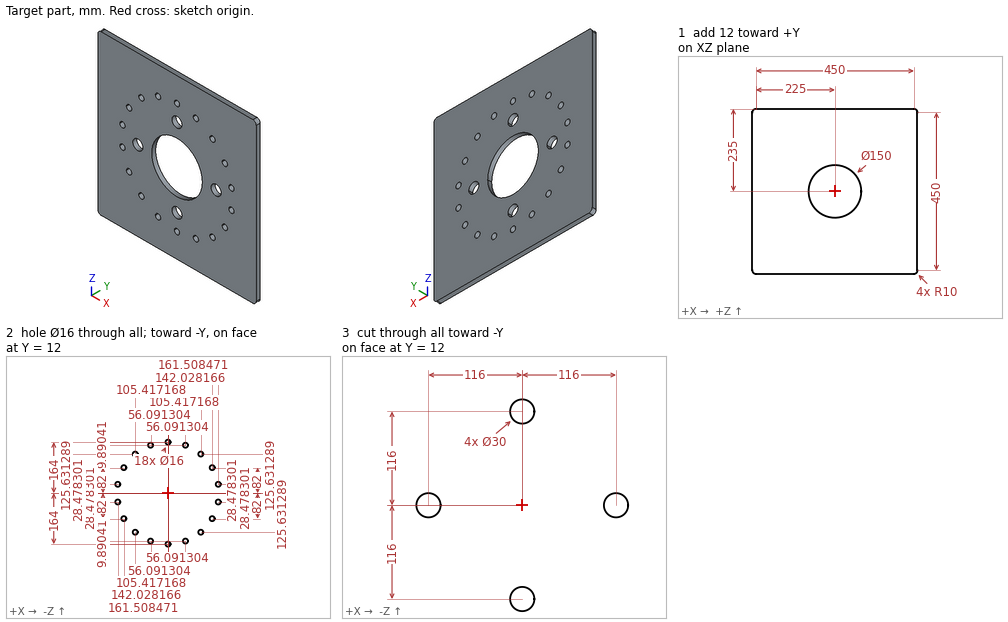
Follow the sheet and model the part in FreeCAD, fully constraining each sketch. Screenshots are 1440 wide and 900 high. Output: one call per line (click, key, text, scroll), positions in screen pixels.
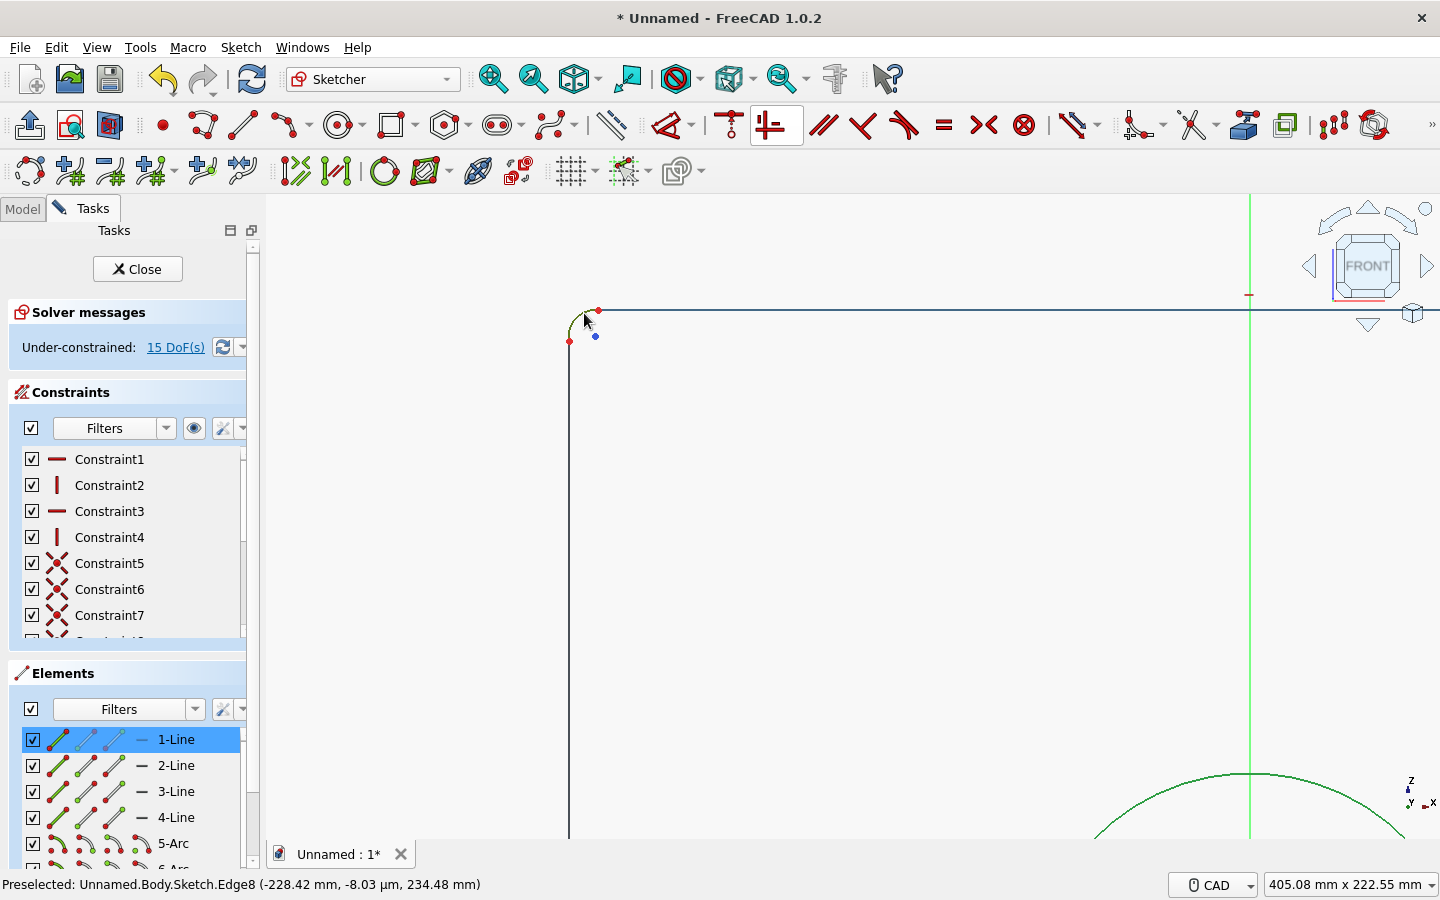
key(t)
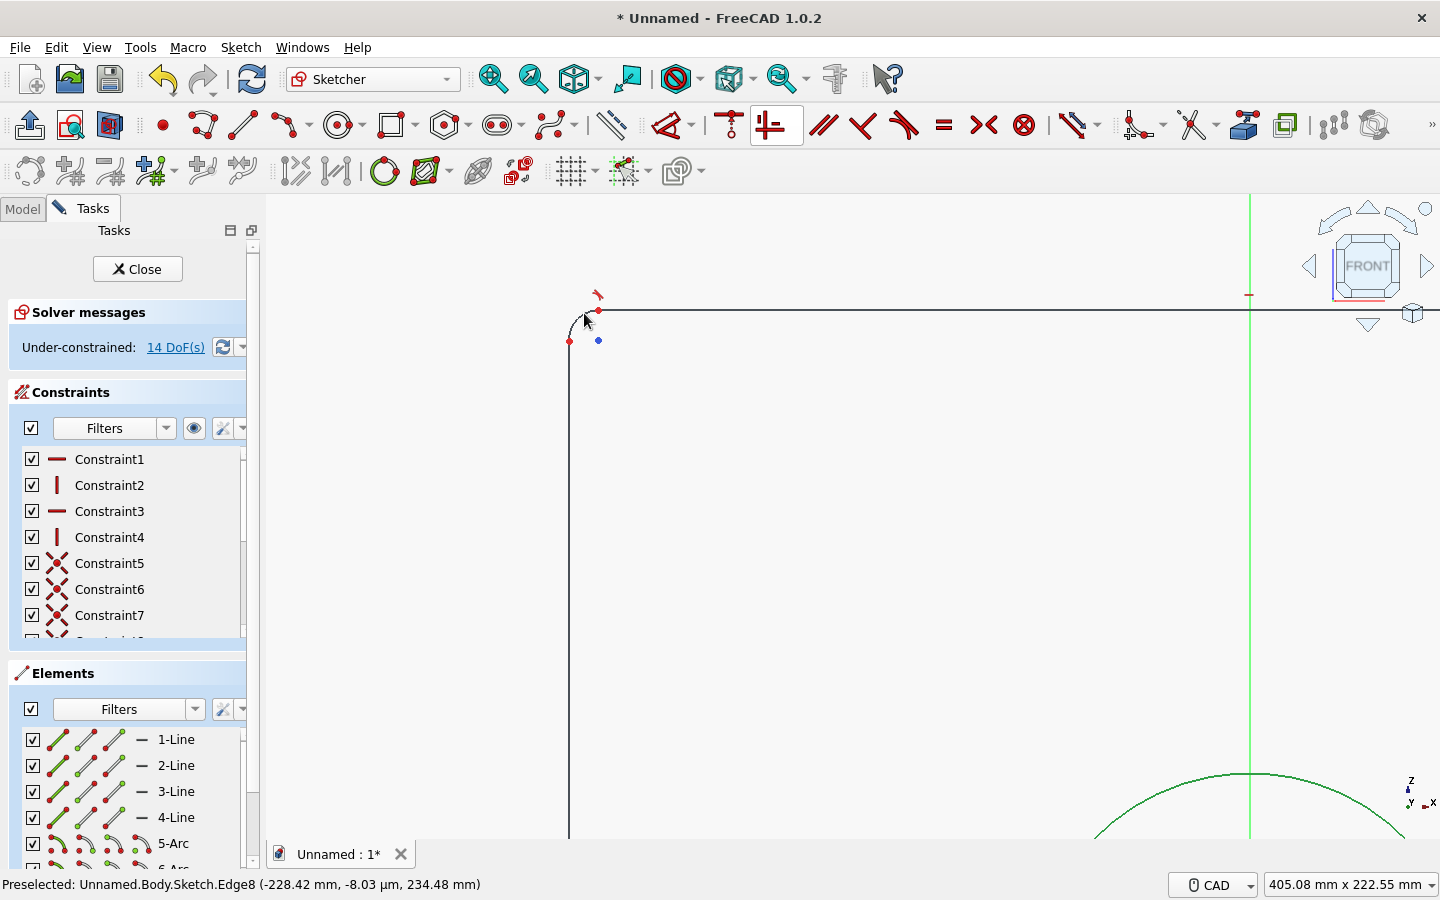
scroll(584, 312, down, 6)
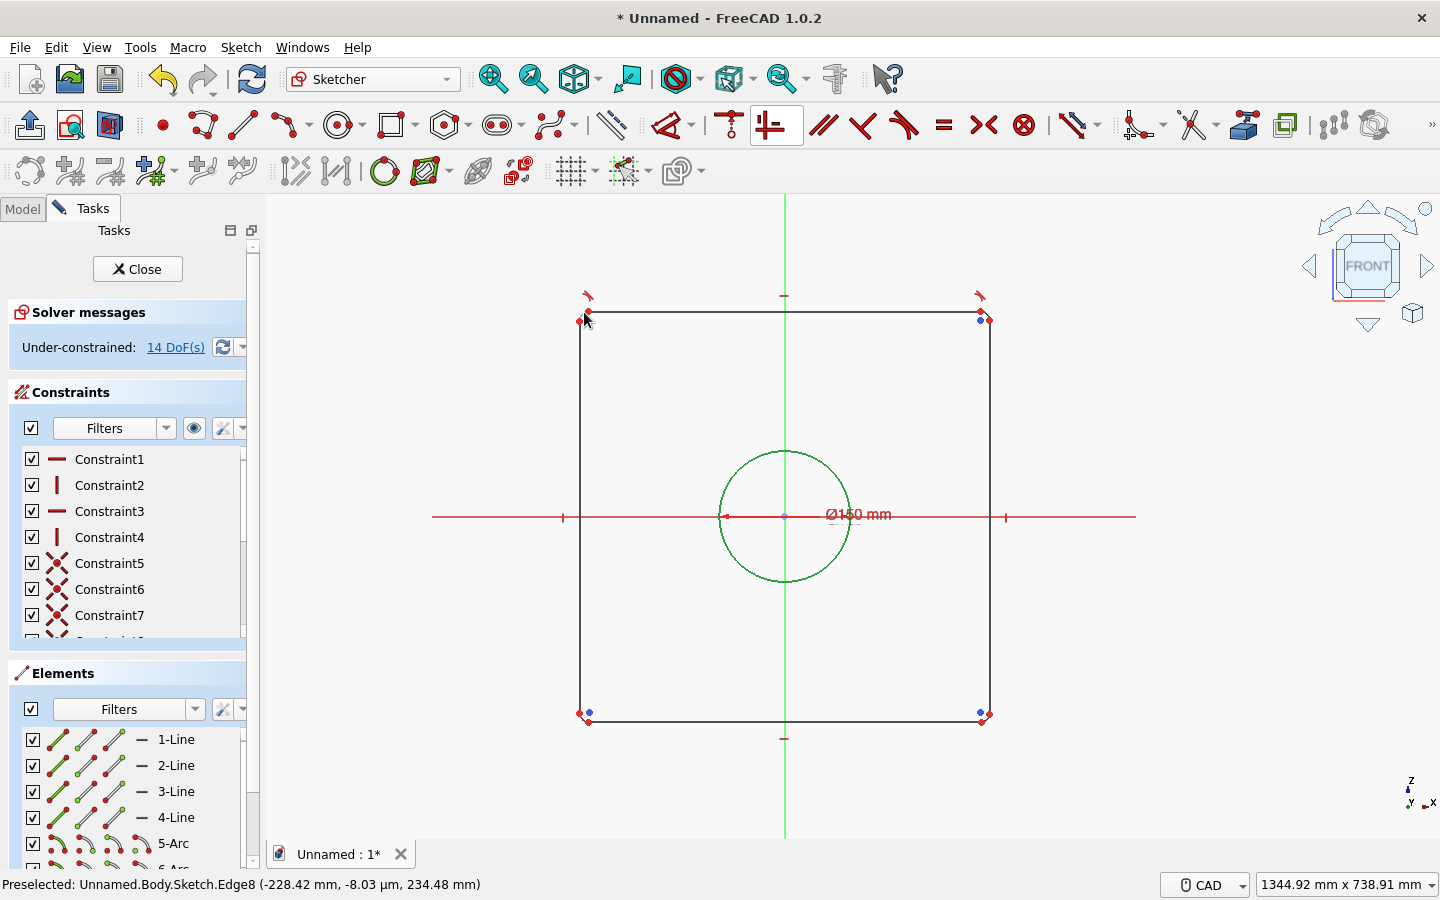
click(990, 439)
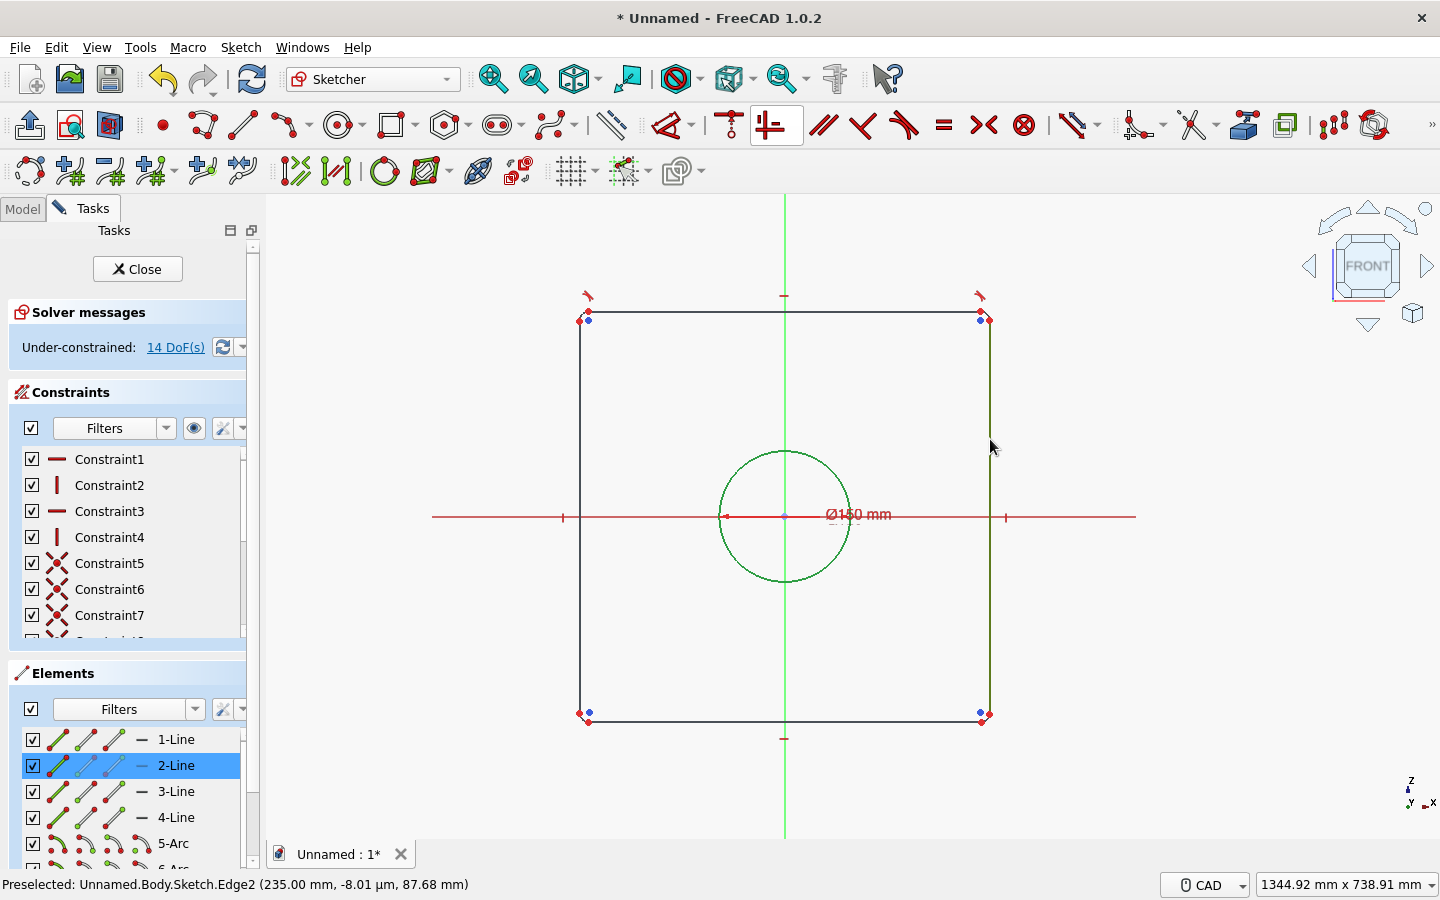
scroll(987, 314, up, 4)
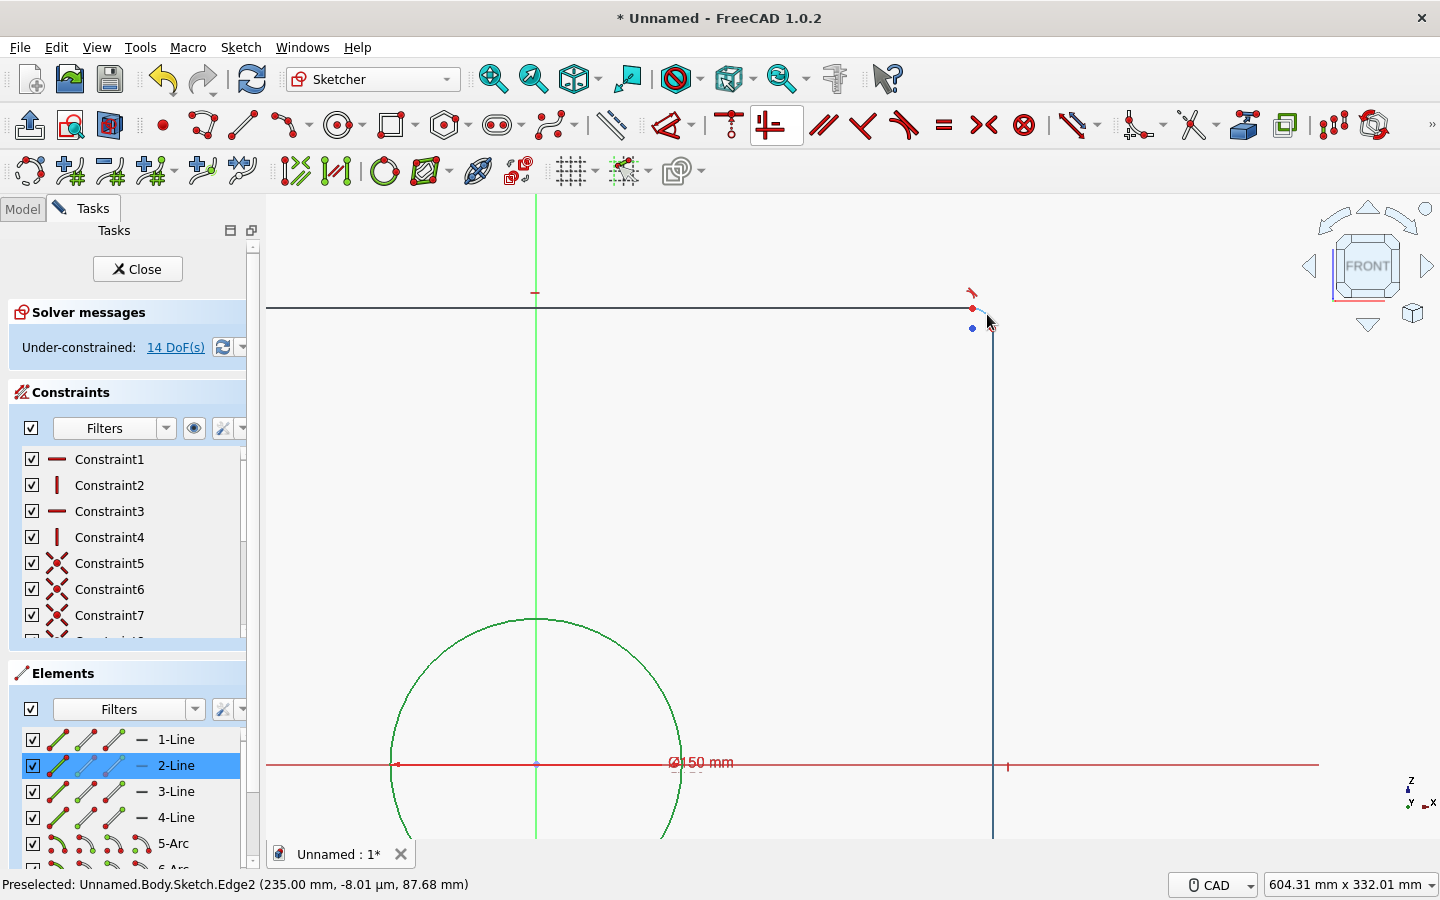
click(987, 314)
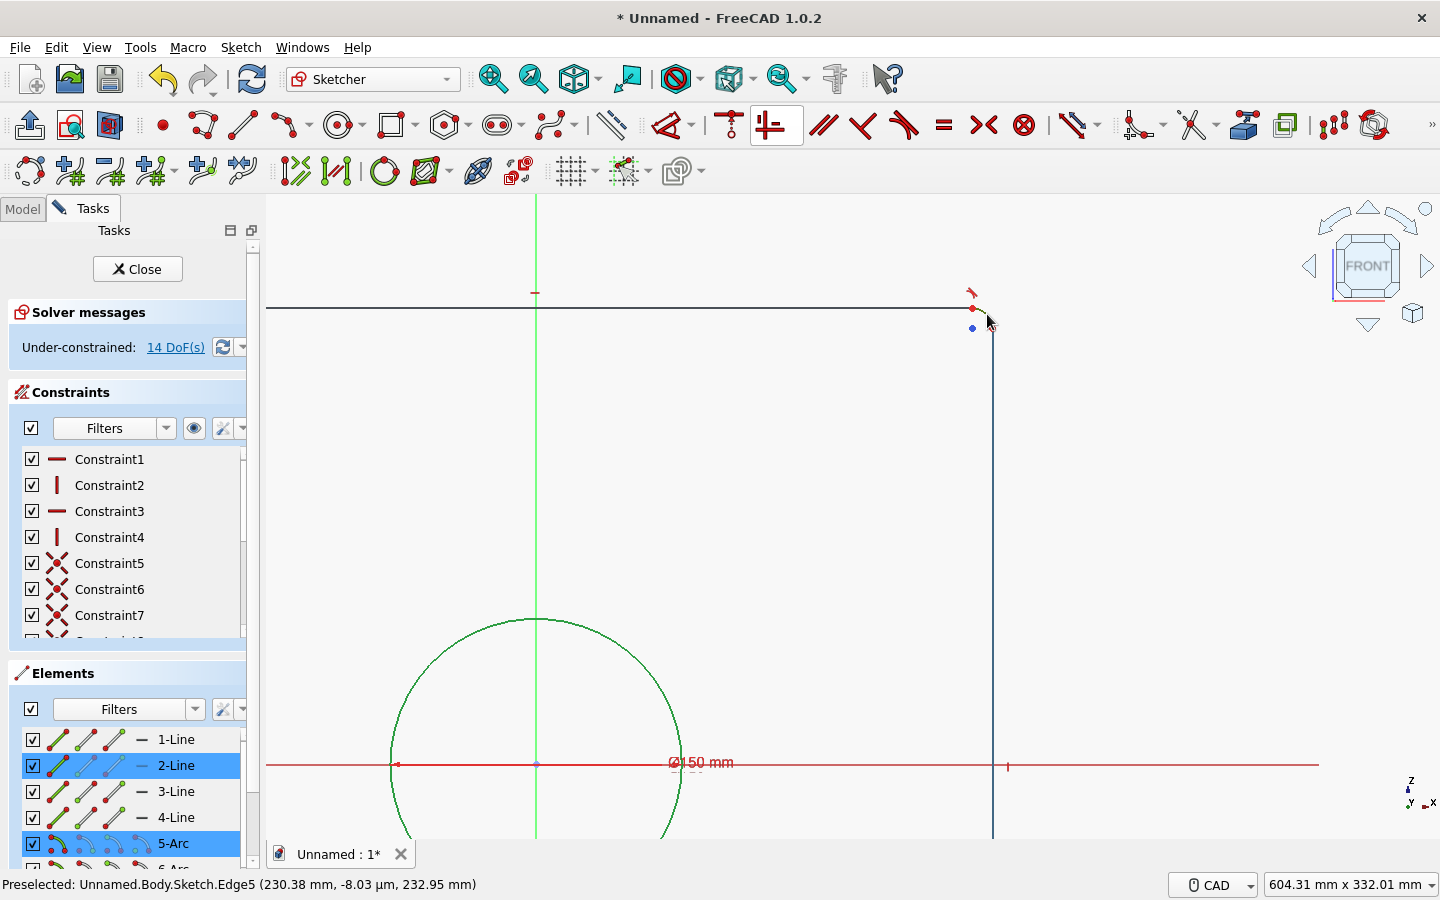
key(t)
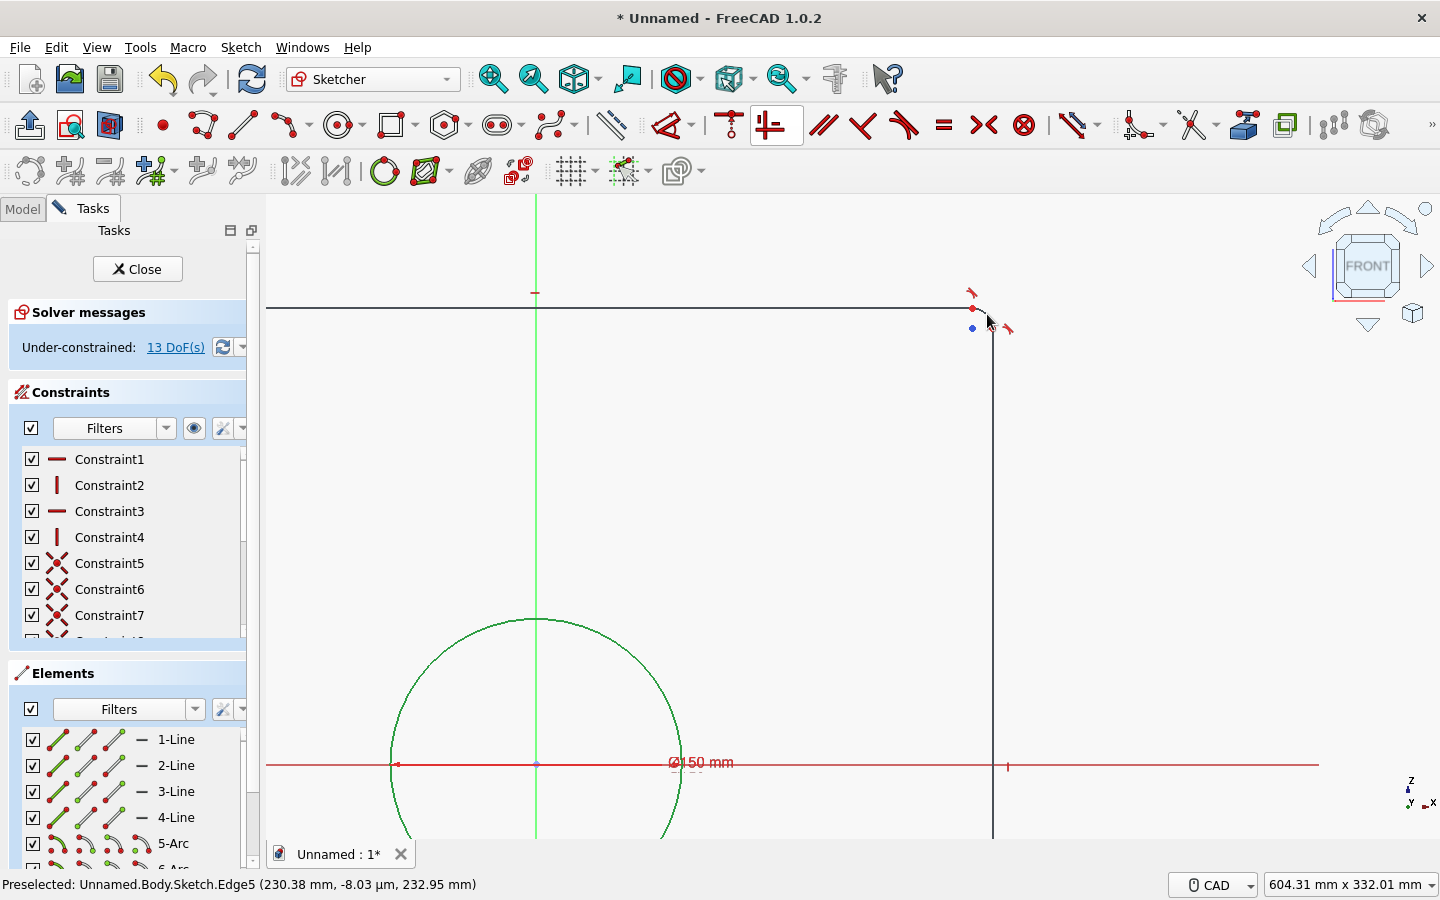
click(993, 591)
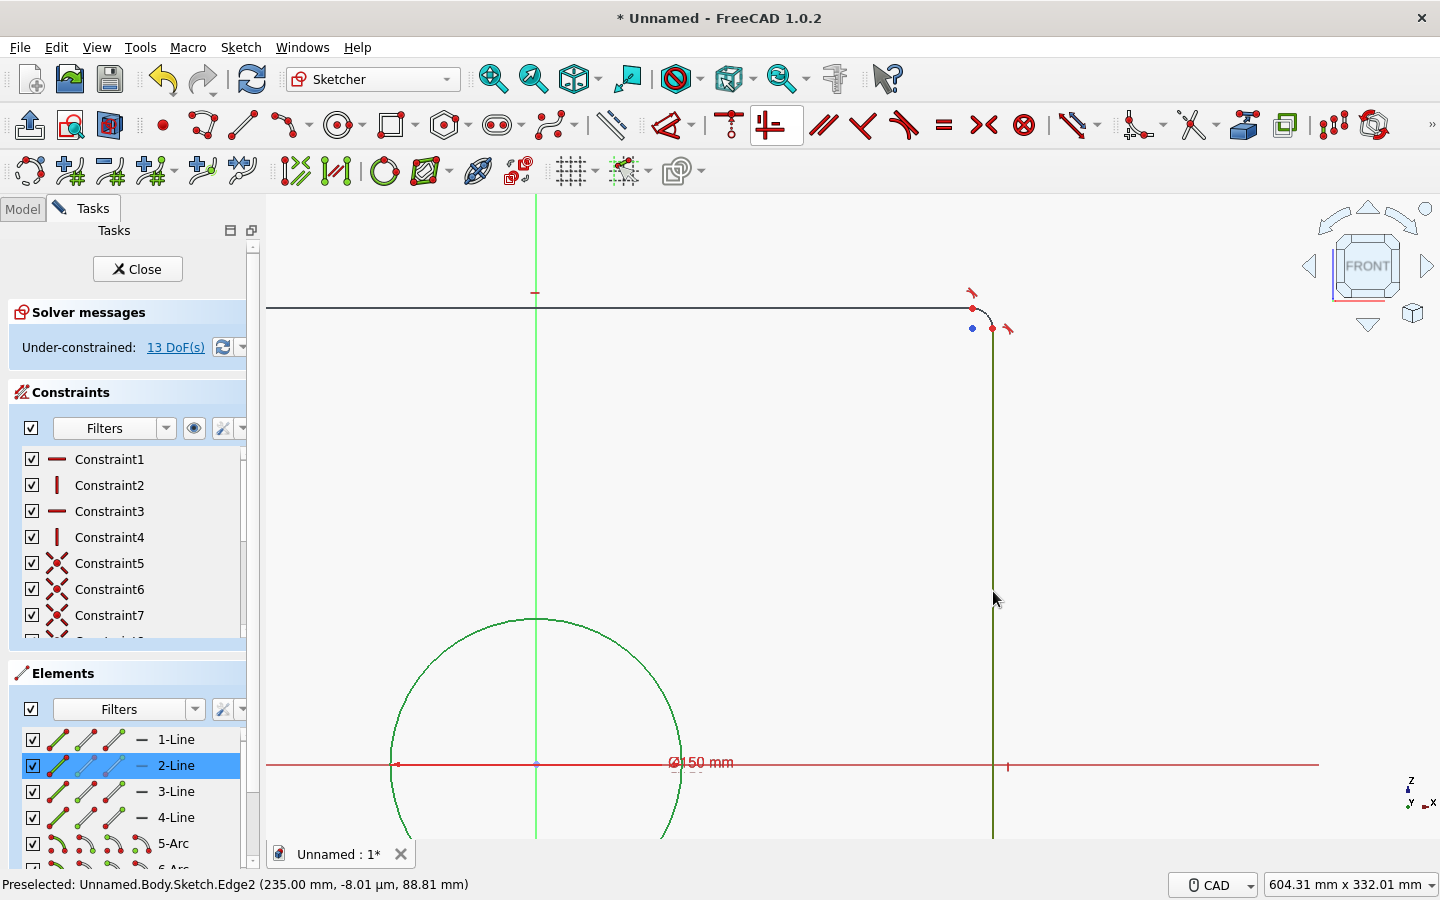
scroll(987, 314, down, 4)